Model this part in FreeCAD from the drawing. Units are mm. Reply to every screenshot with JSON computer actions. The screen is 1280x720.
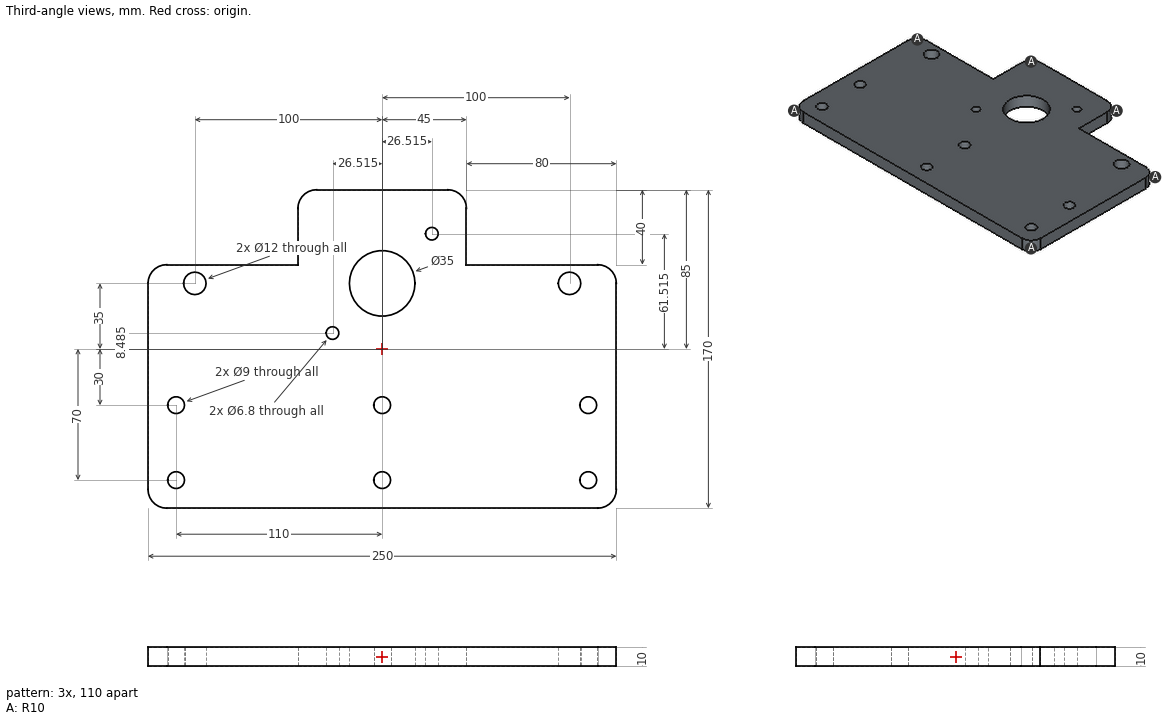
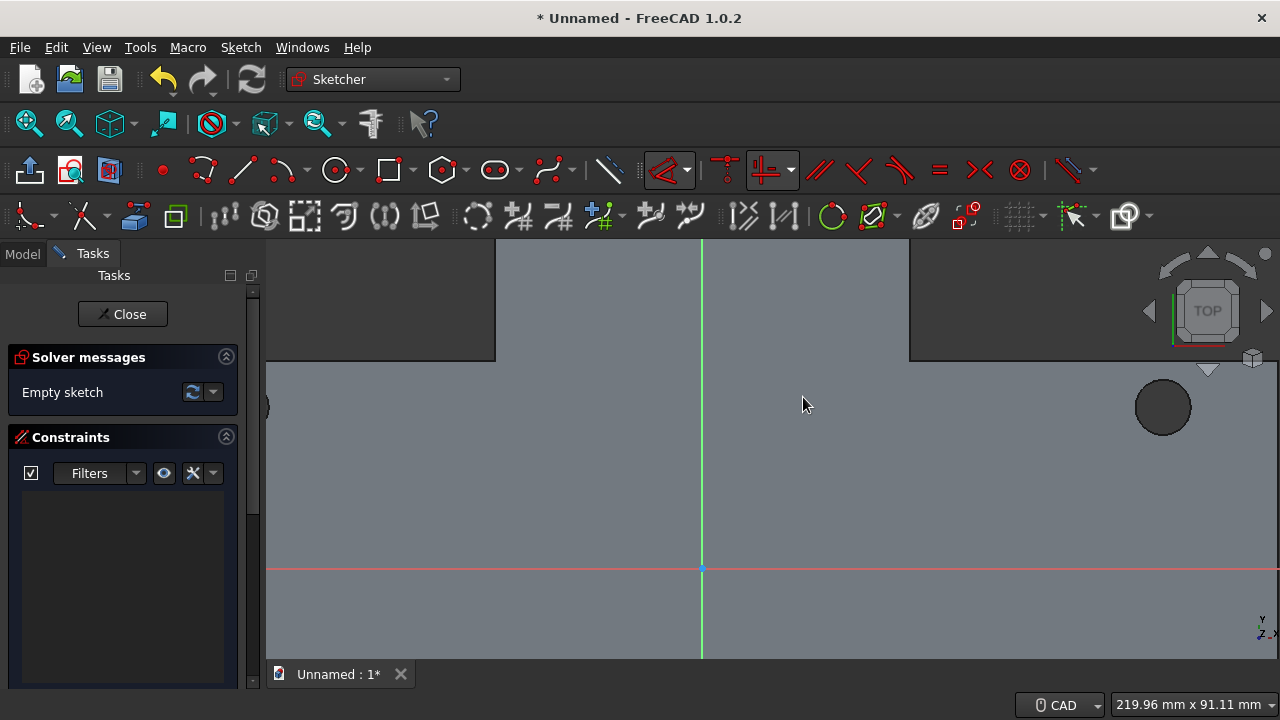
{"action": "left_click", "coordinate": [336, 170]}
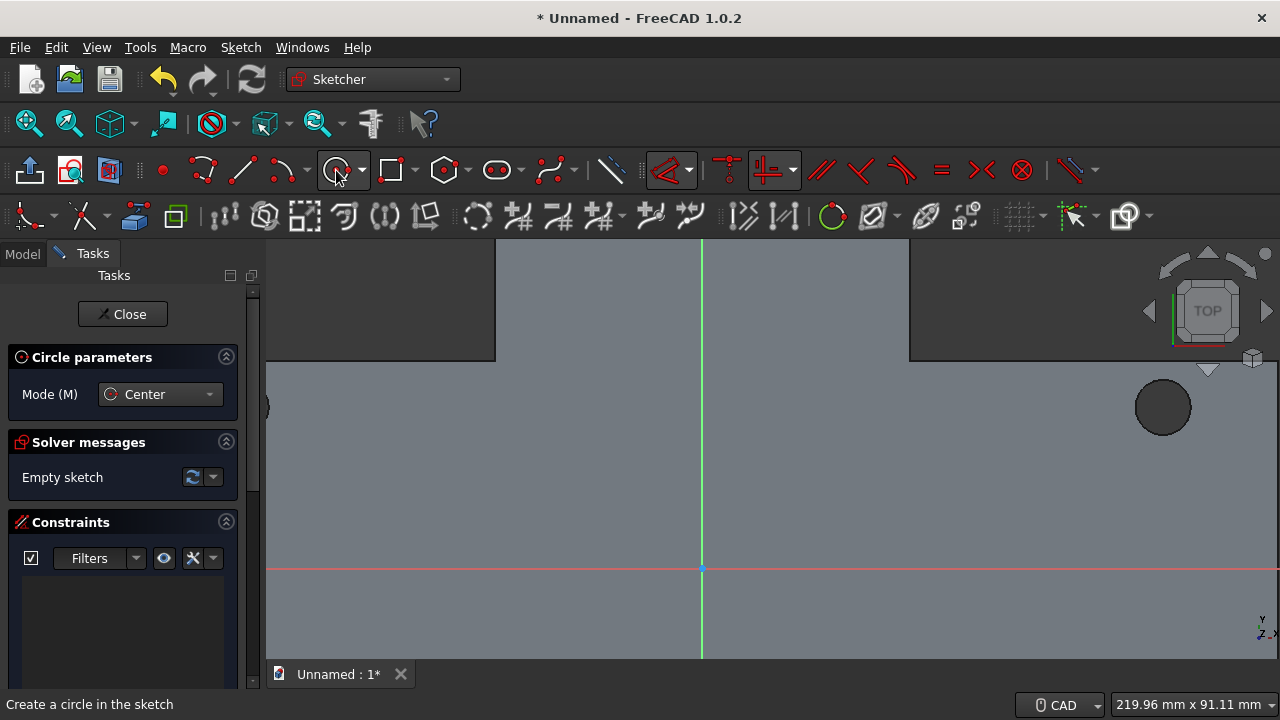
{"action": "left_click", "coordinate": [702, 407]}
{"action": "mouse_move", "coordinate": [759, 350]}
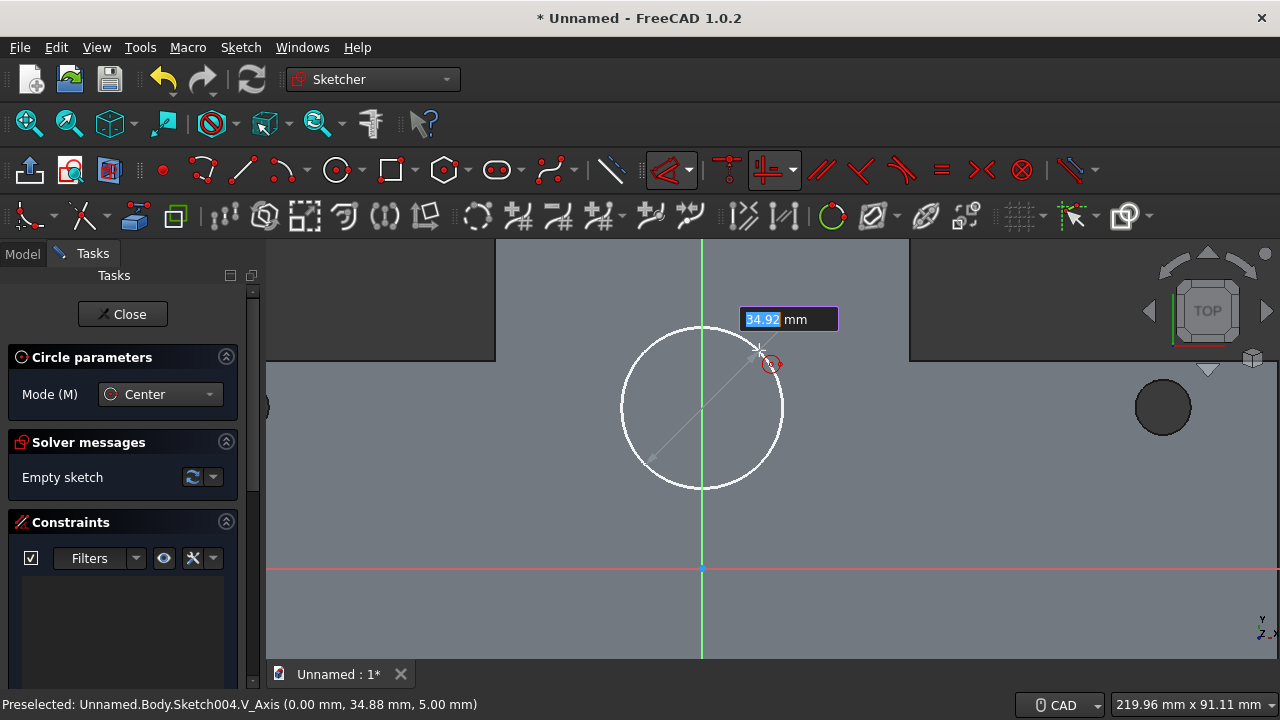
{"action": "type", "text": "35"}
{"action": "key", "text": "Return"}
{"action": "key", "text": "Escape"}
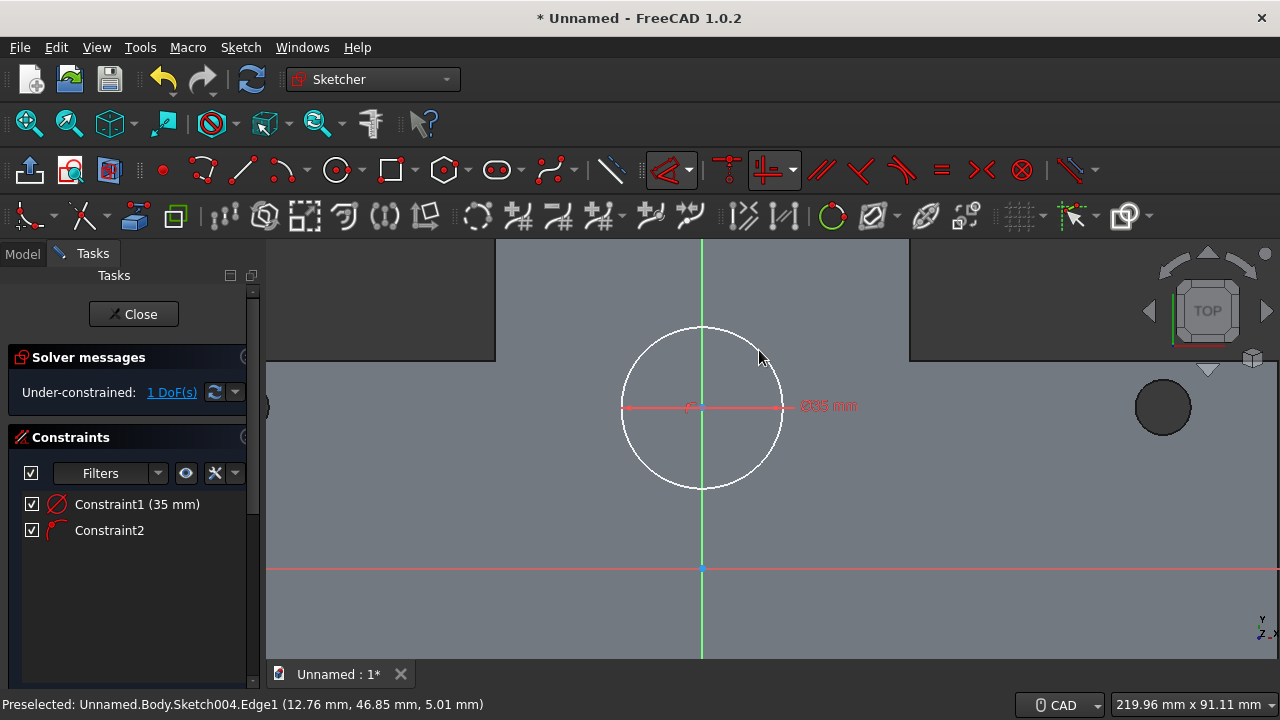
{"action": "left_click", "coordinate": [702, 408]}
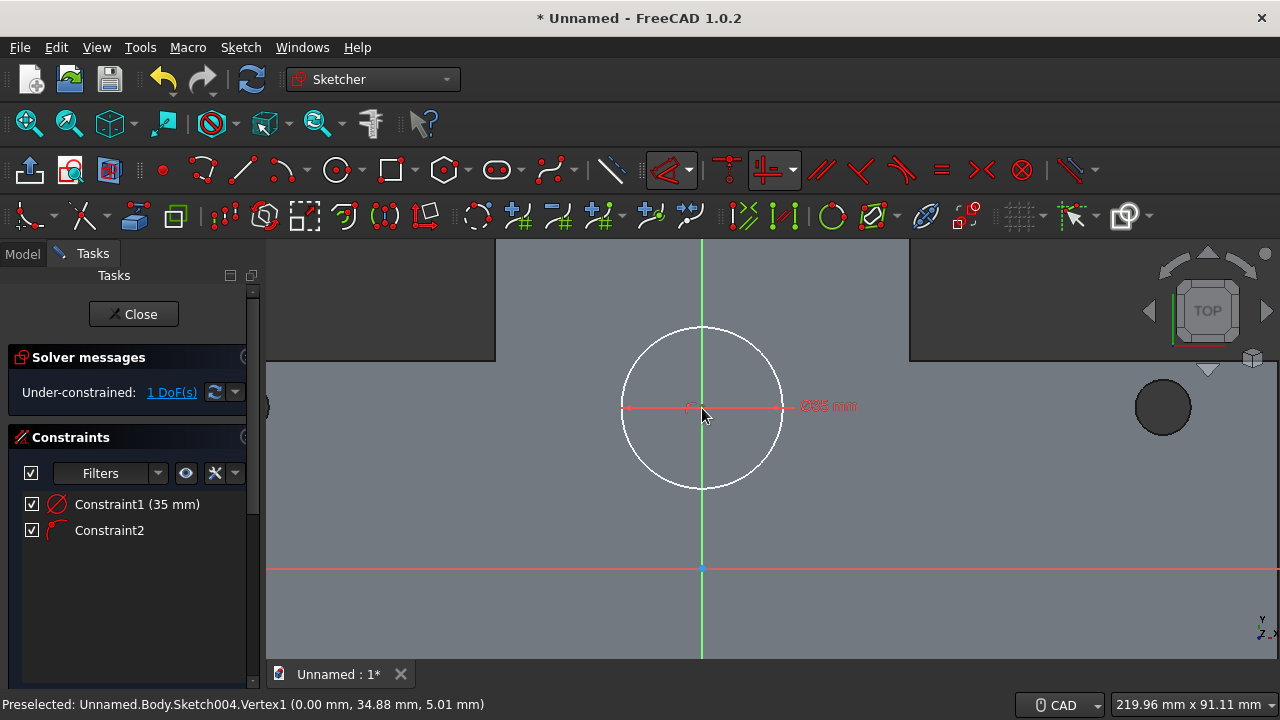
{"action": "left_click", "coordinate": [692, 170]}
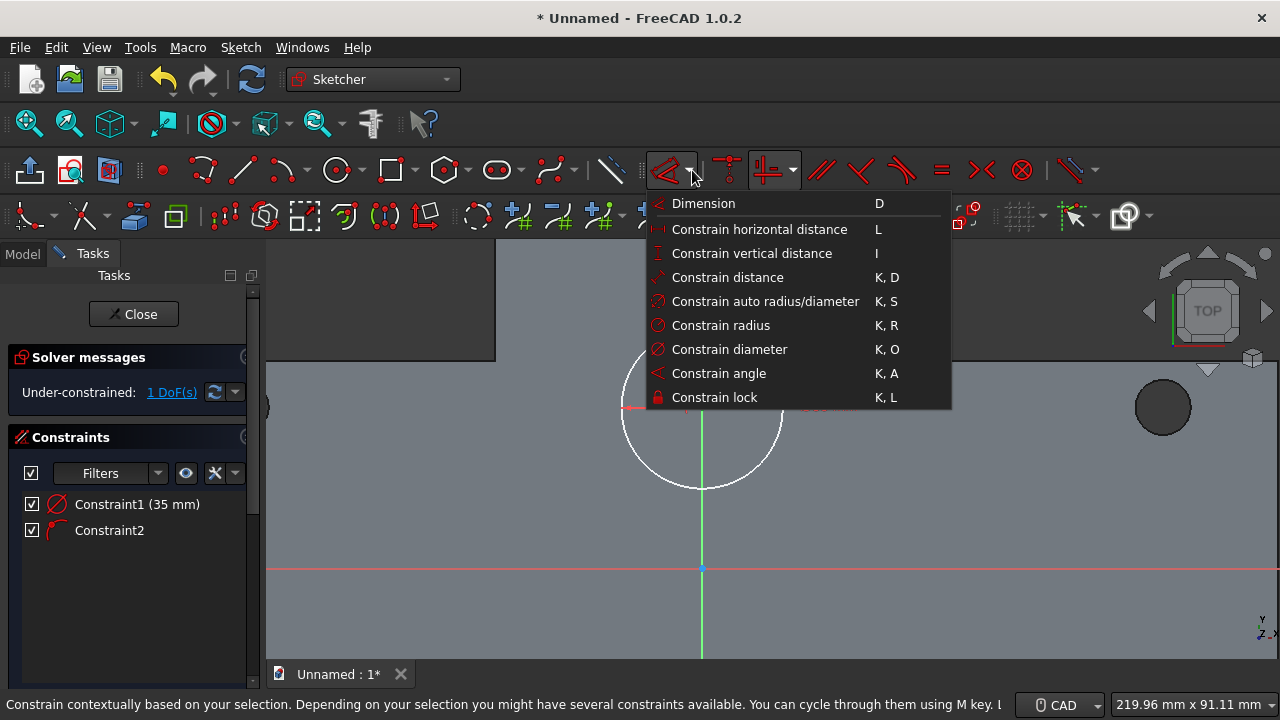
{"action": "left_click", "coordinate": [799, 253]}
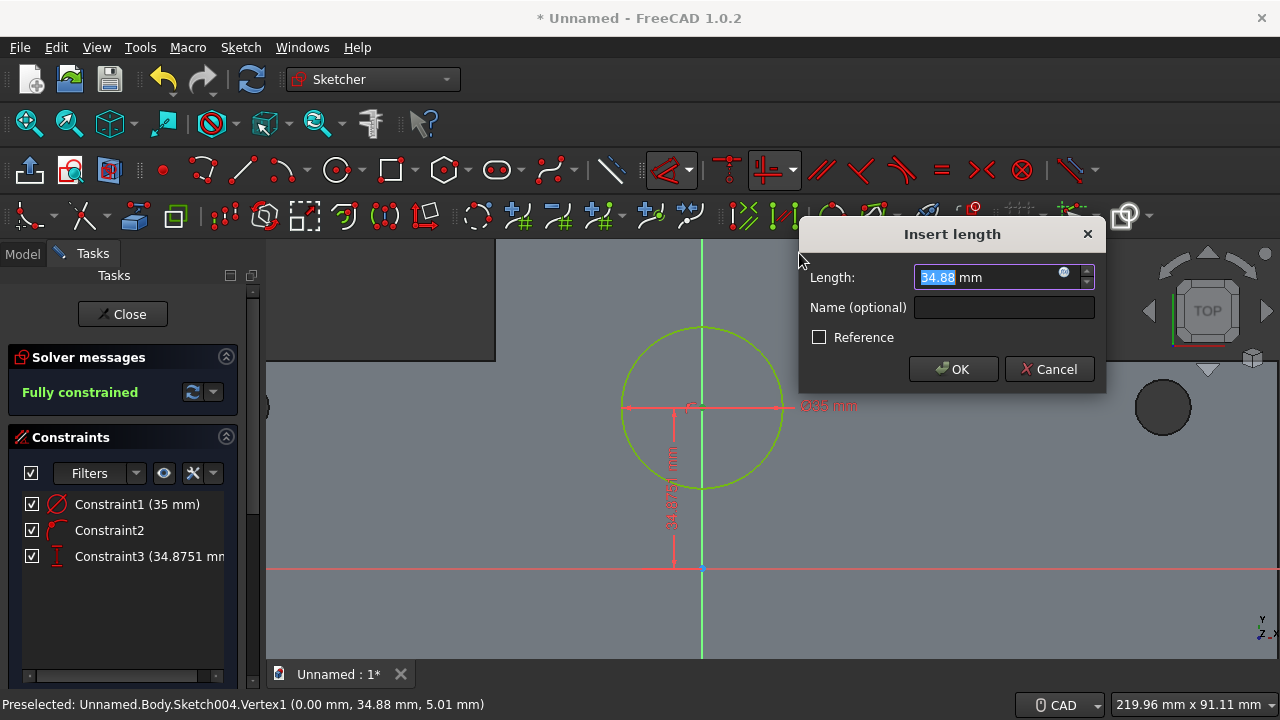
{"action": "type", "text": "35"}
{"action": "key", "text": "Return"}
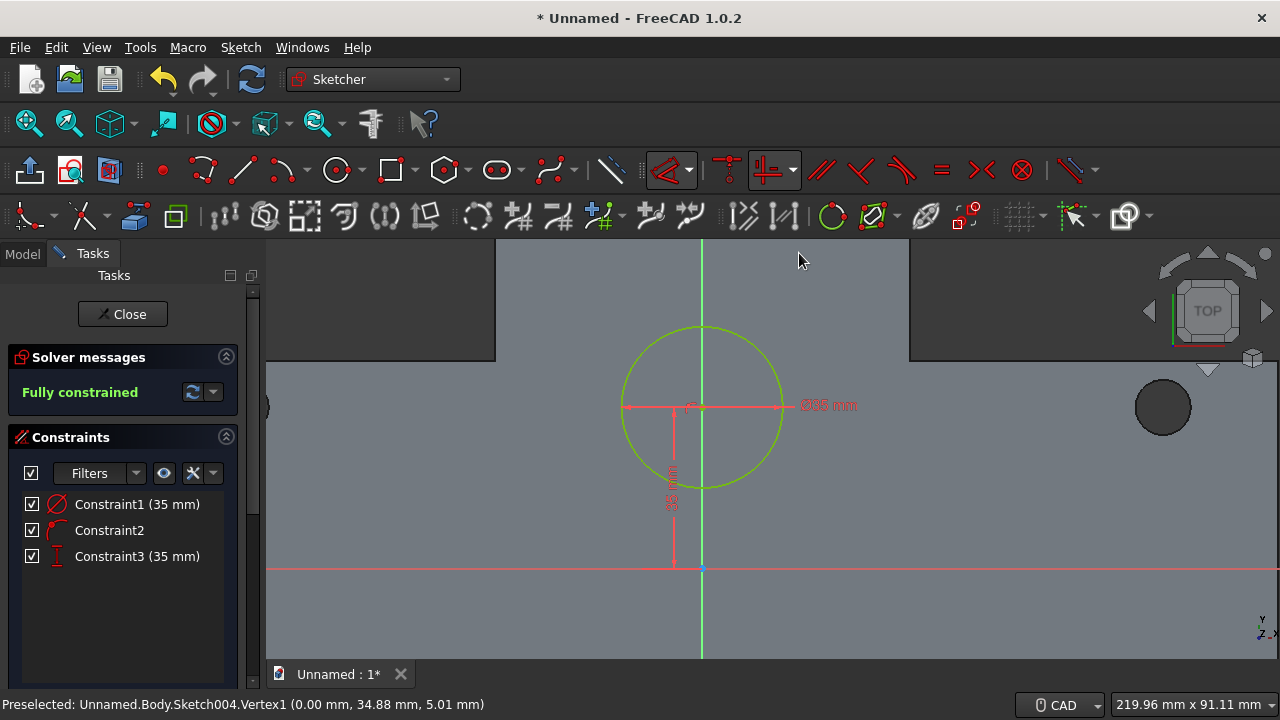
{"action": "left_click", "coordinate": [123, 314]}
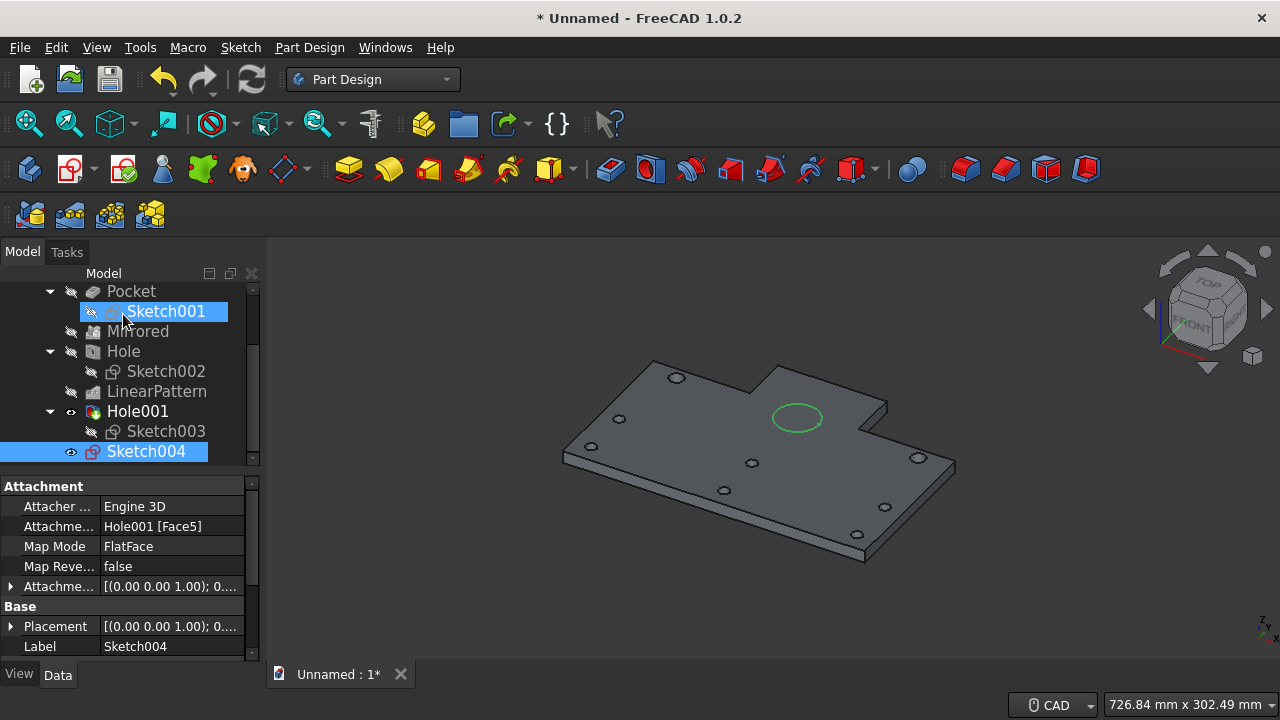
{"action": "left_click", "coordinate": [612, 170]}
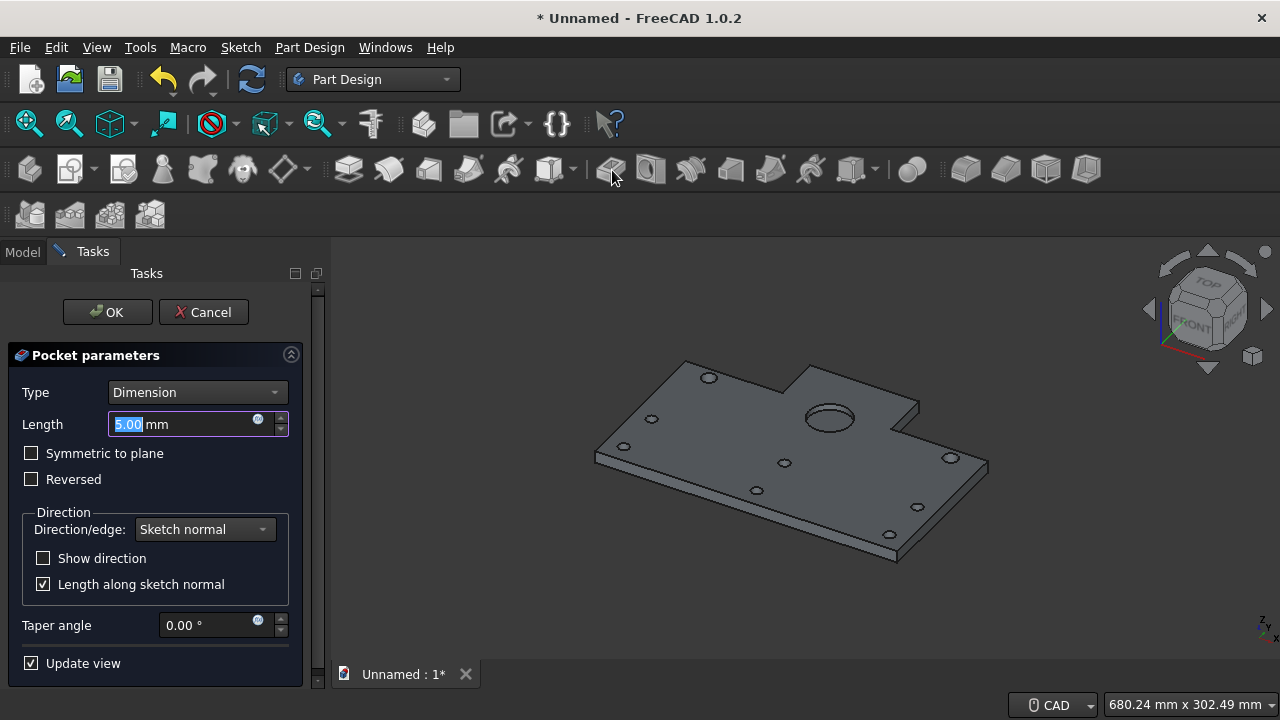
{"action": "type", "text": "10"}
{"action": "key", "text": "Tab"}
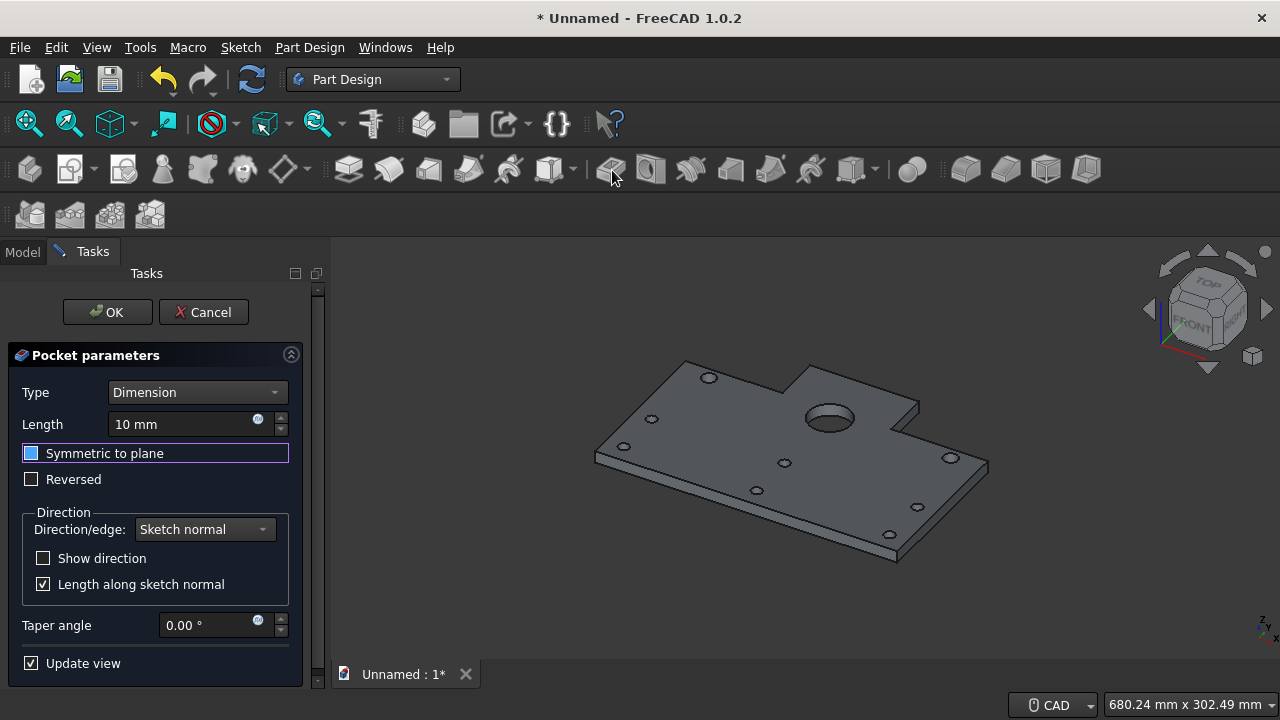
{"action": "left_click", "coordinate": [108, 312]}